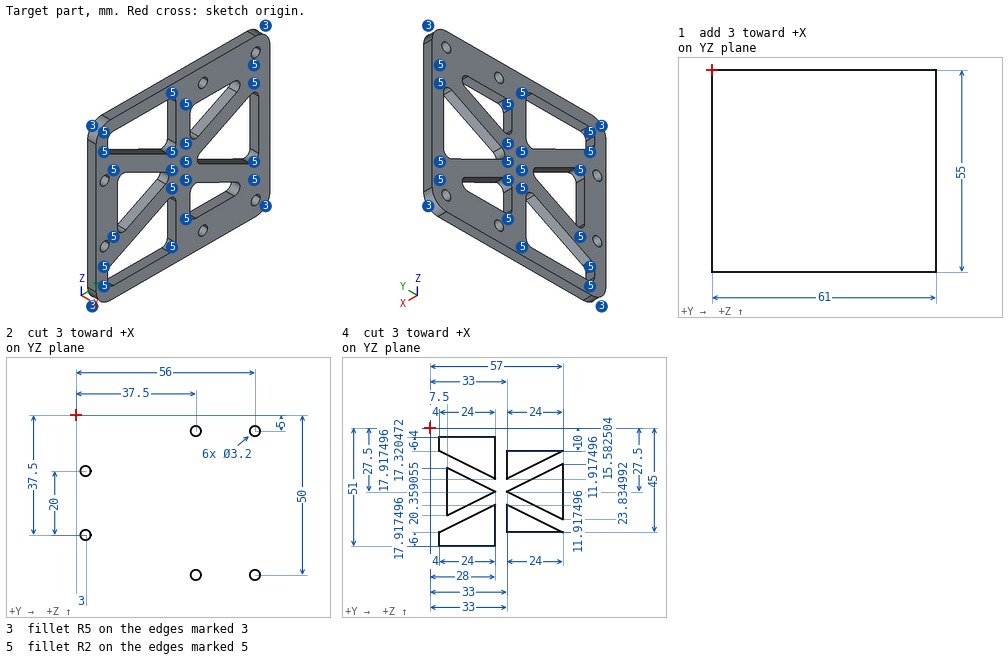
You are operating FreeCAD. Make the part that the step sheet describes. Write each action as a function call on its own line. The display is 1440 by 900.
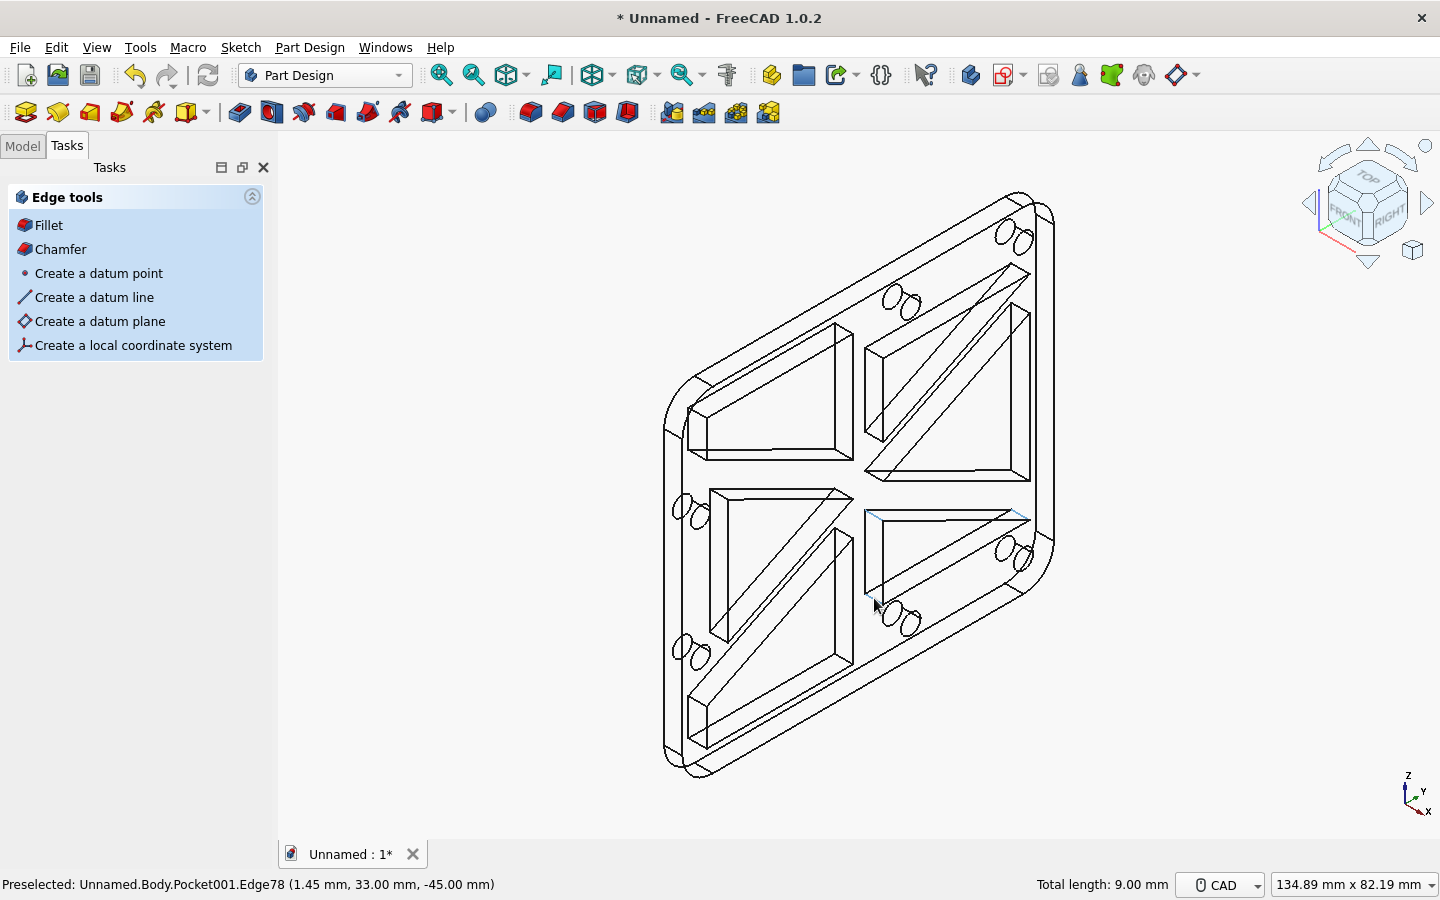
click(1017, 473, ctrl)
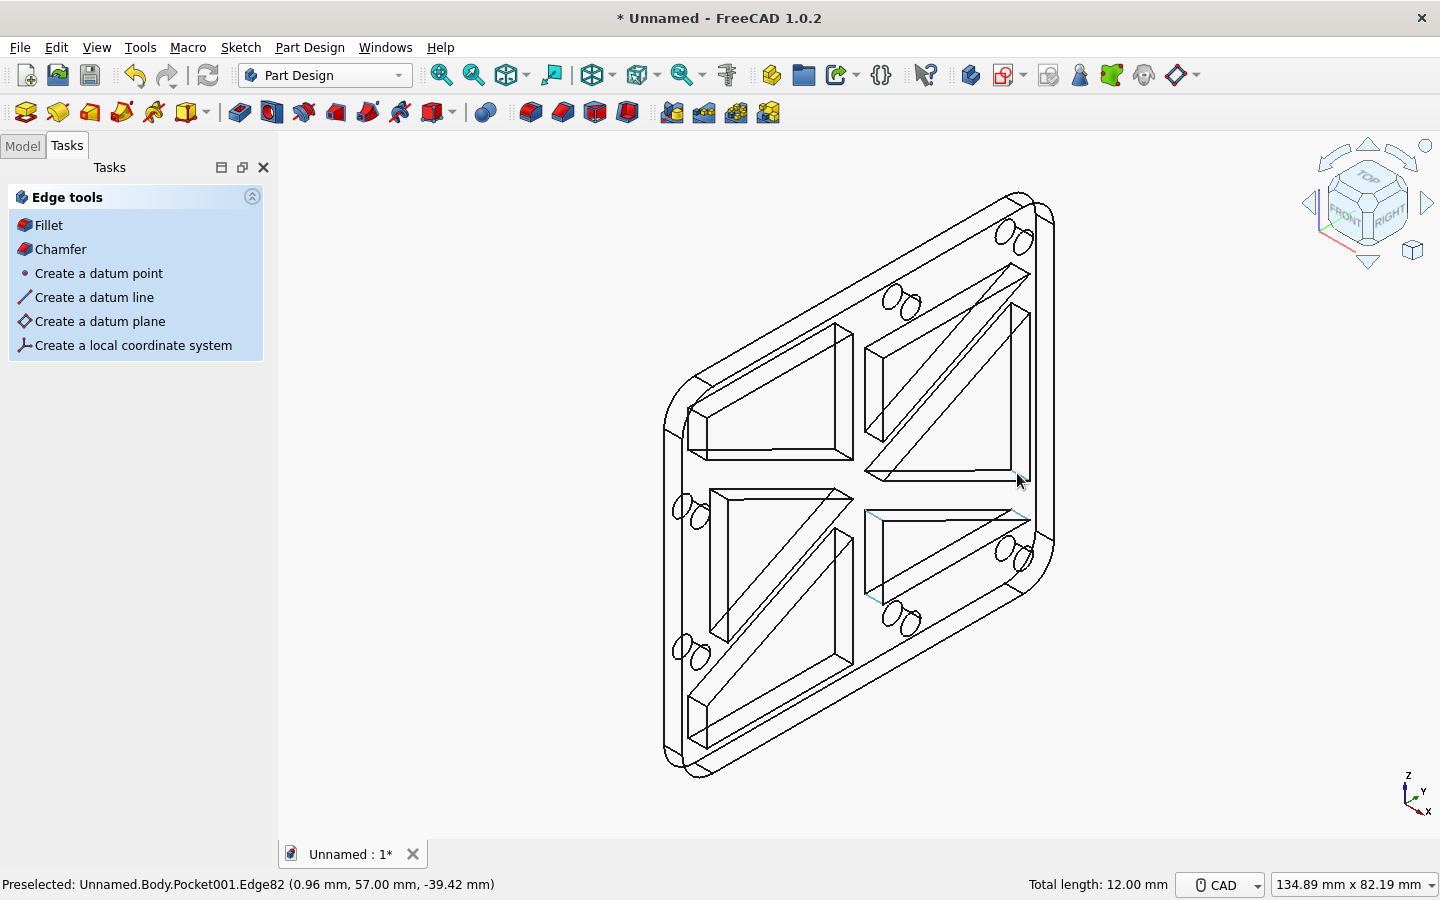
click(1020, 307, ctrl)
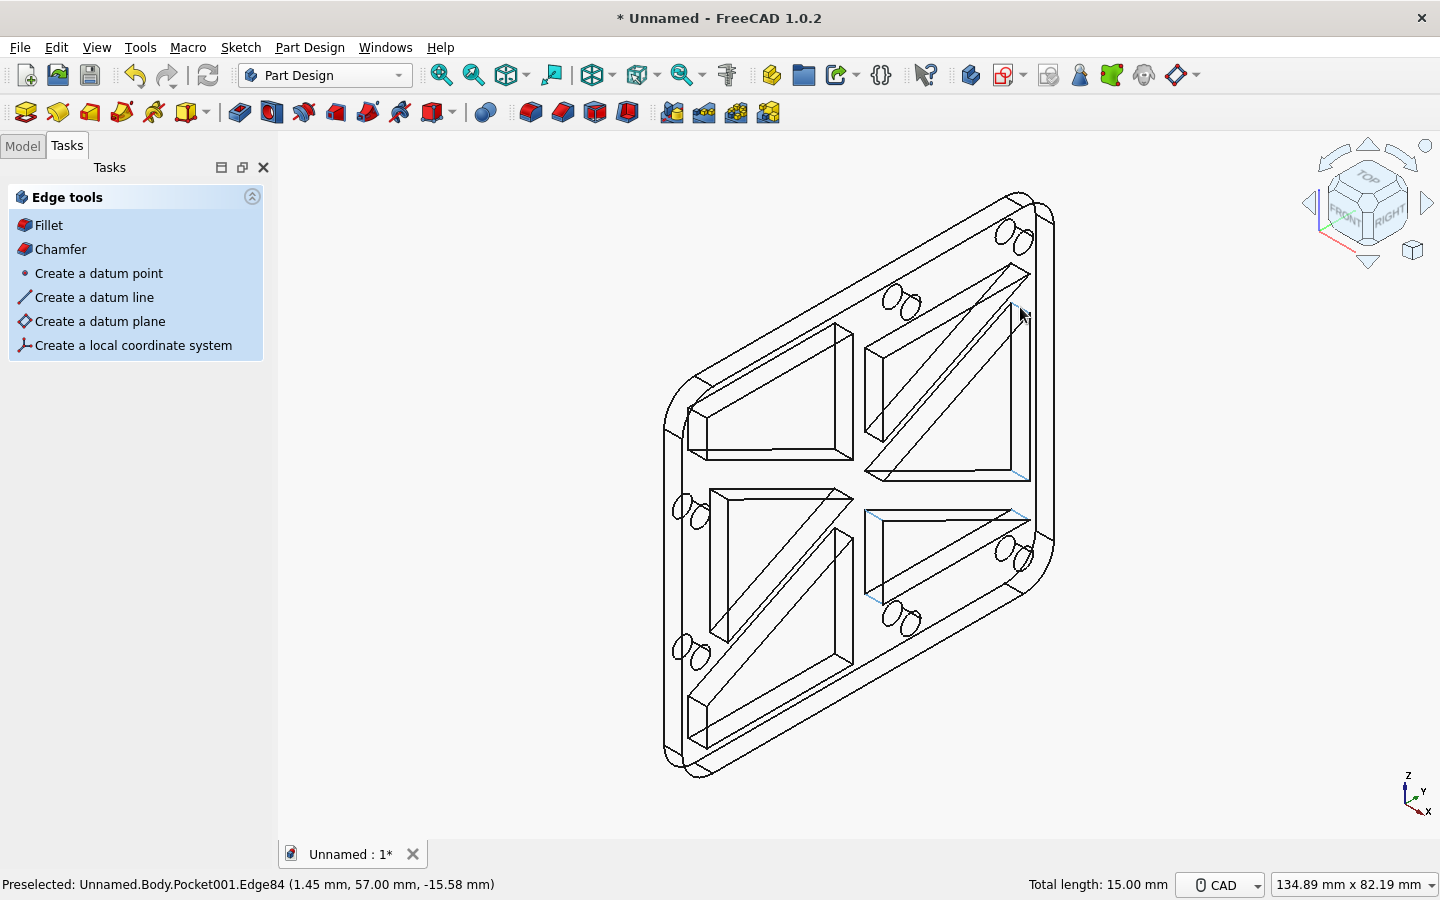
click(874, 475, ctrl)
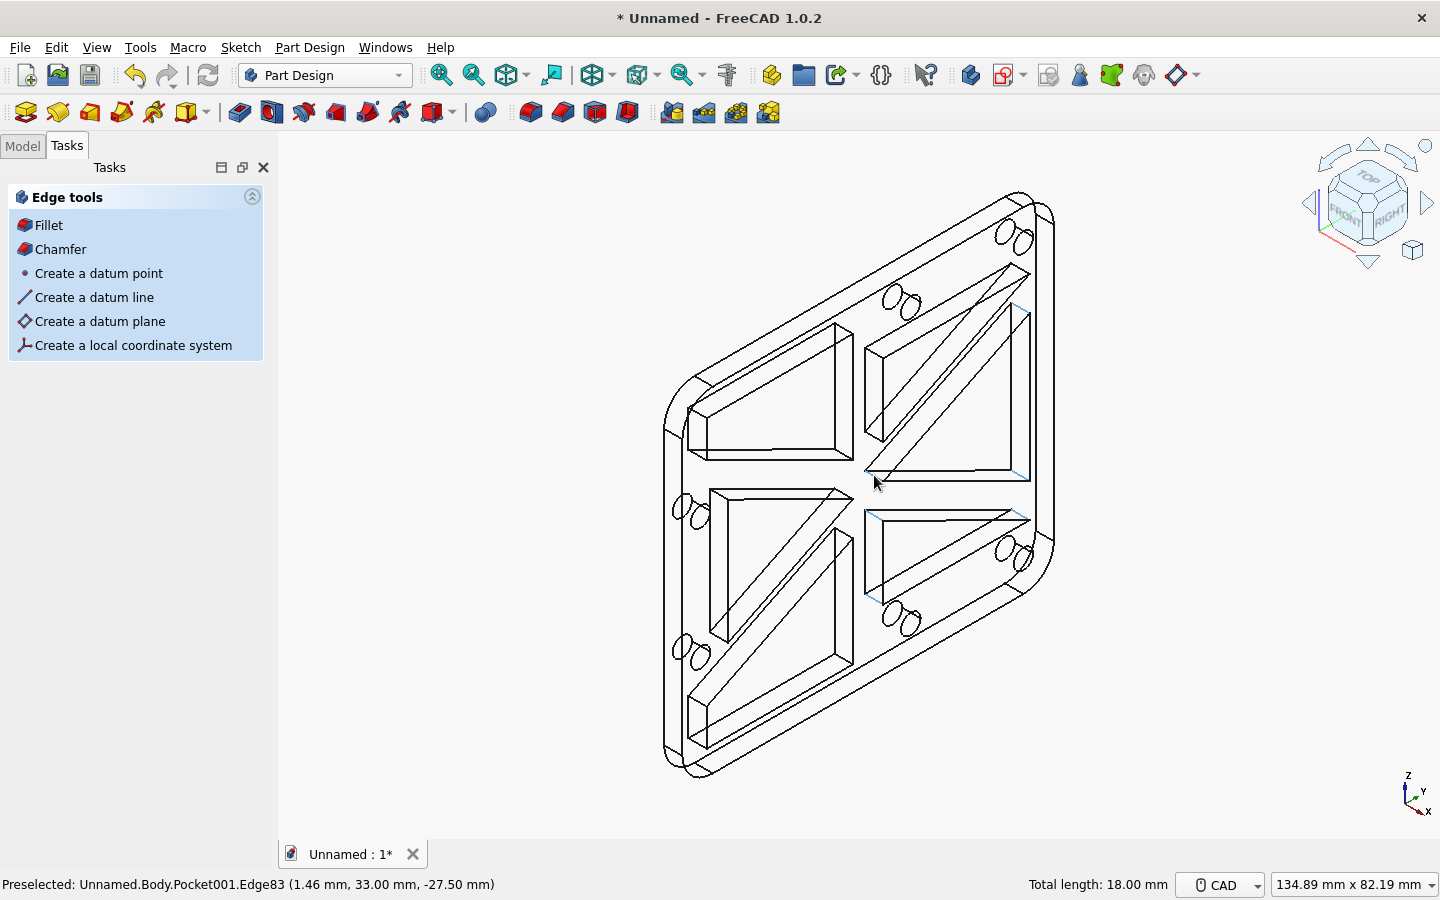
click(842, 492, ctrl)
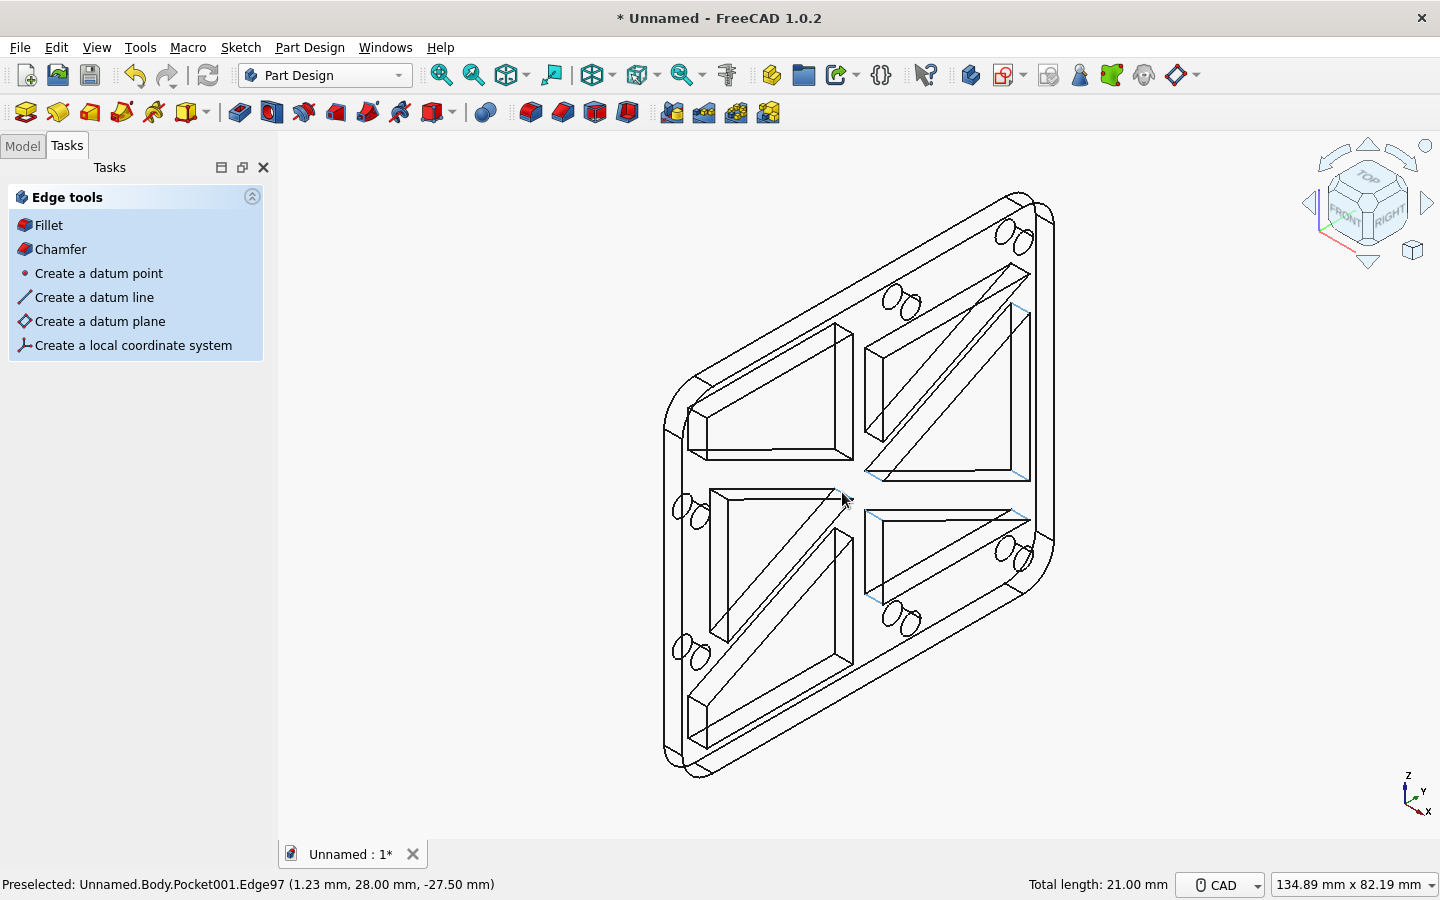
click(719, 493, ctrl)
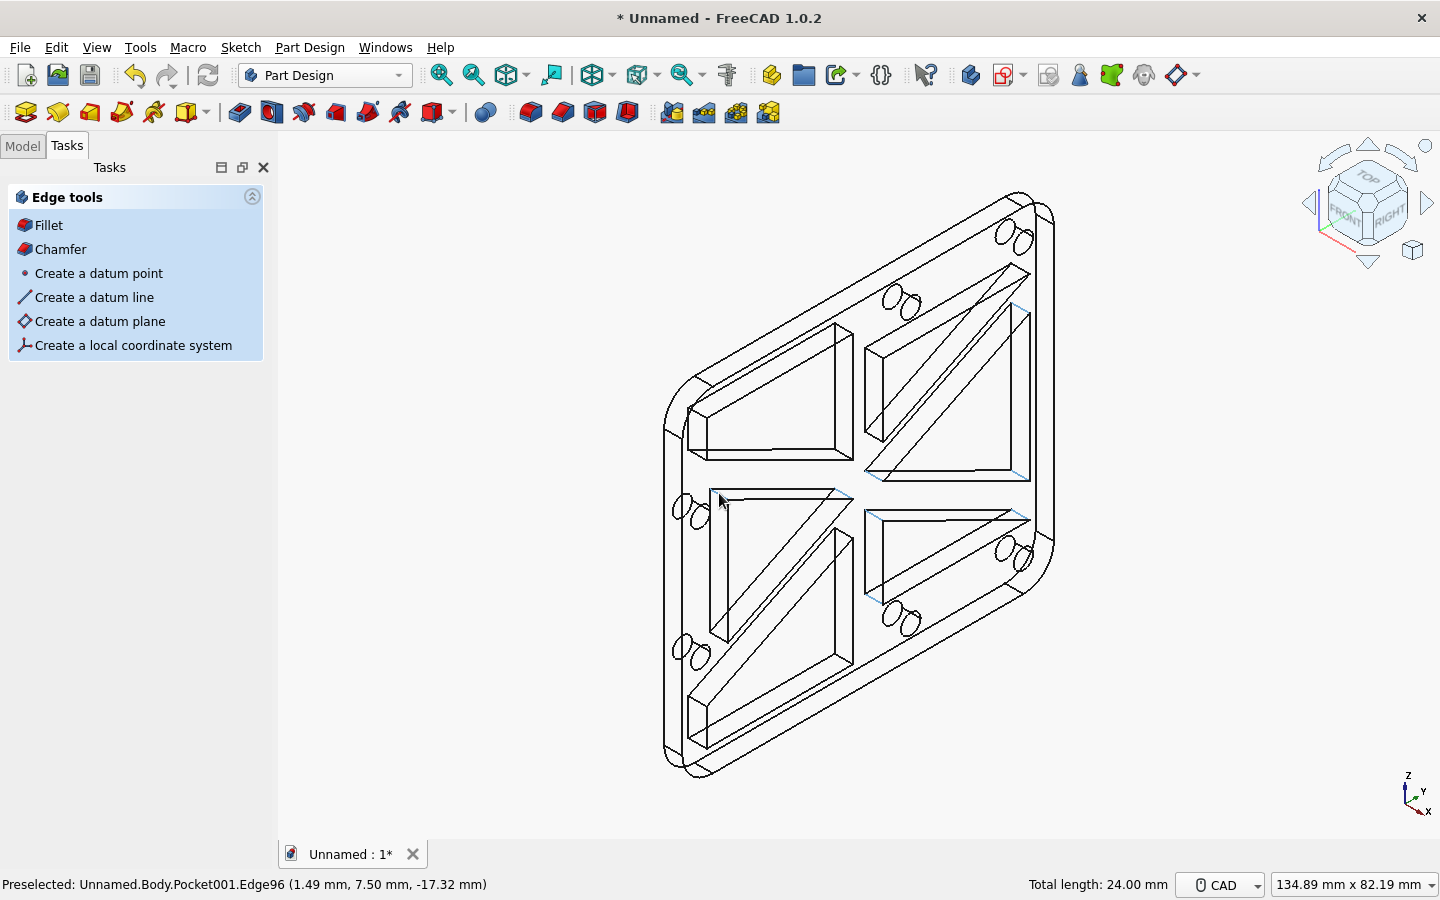
click(719, 636, ctrl)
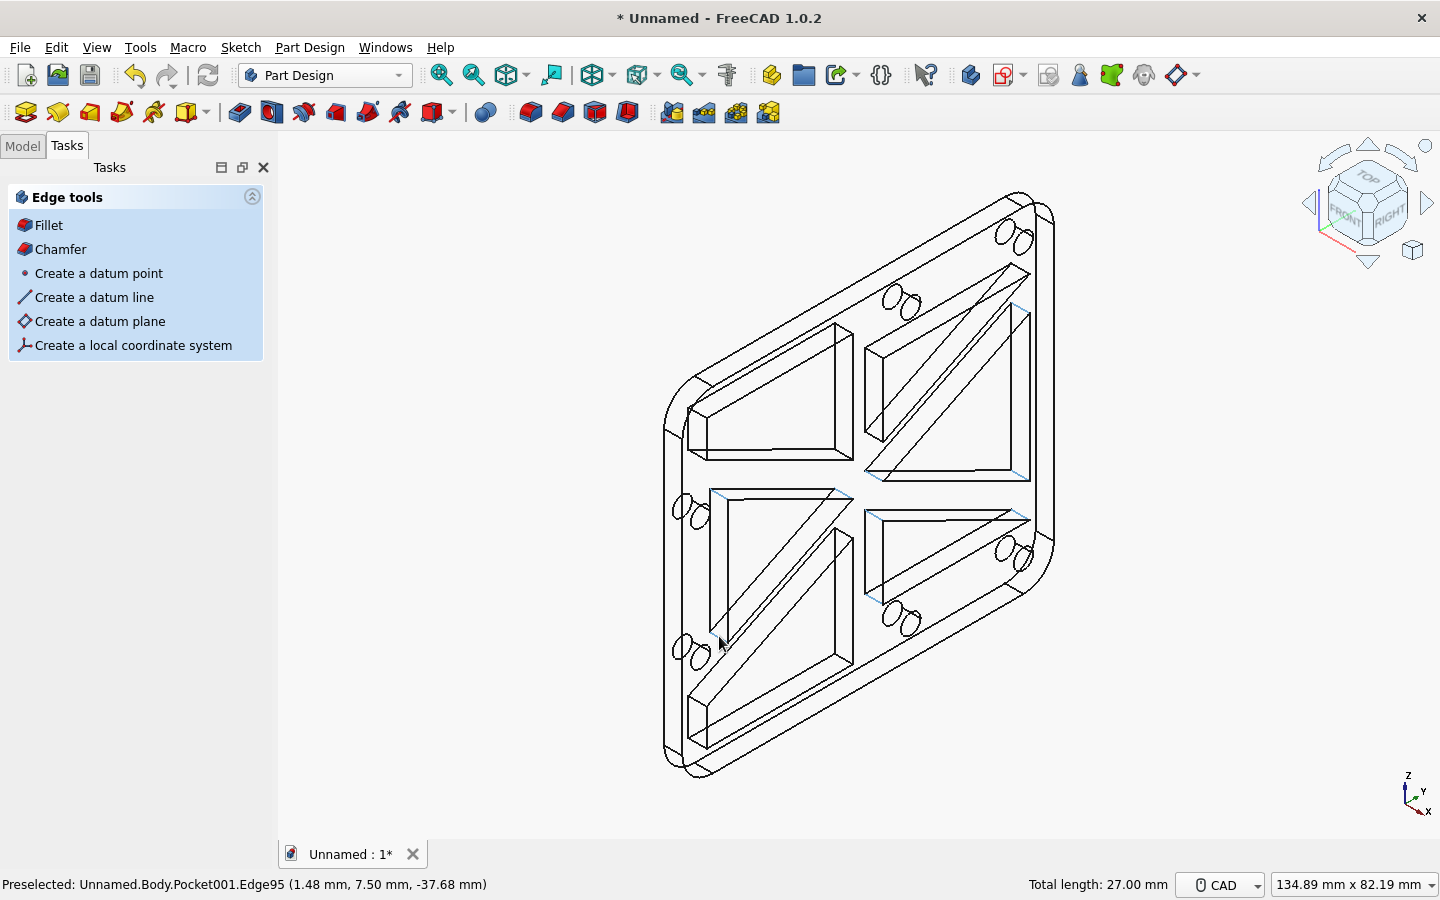
click(844, 328, ctrl)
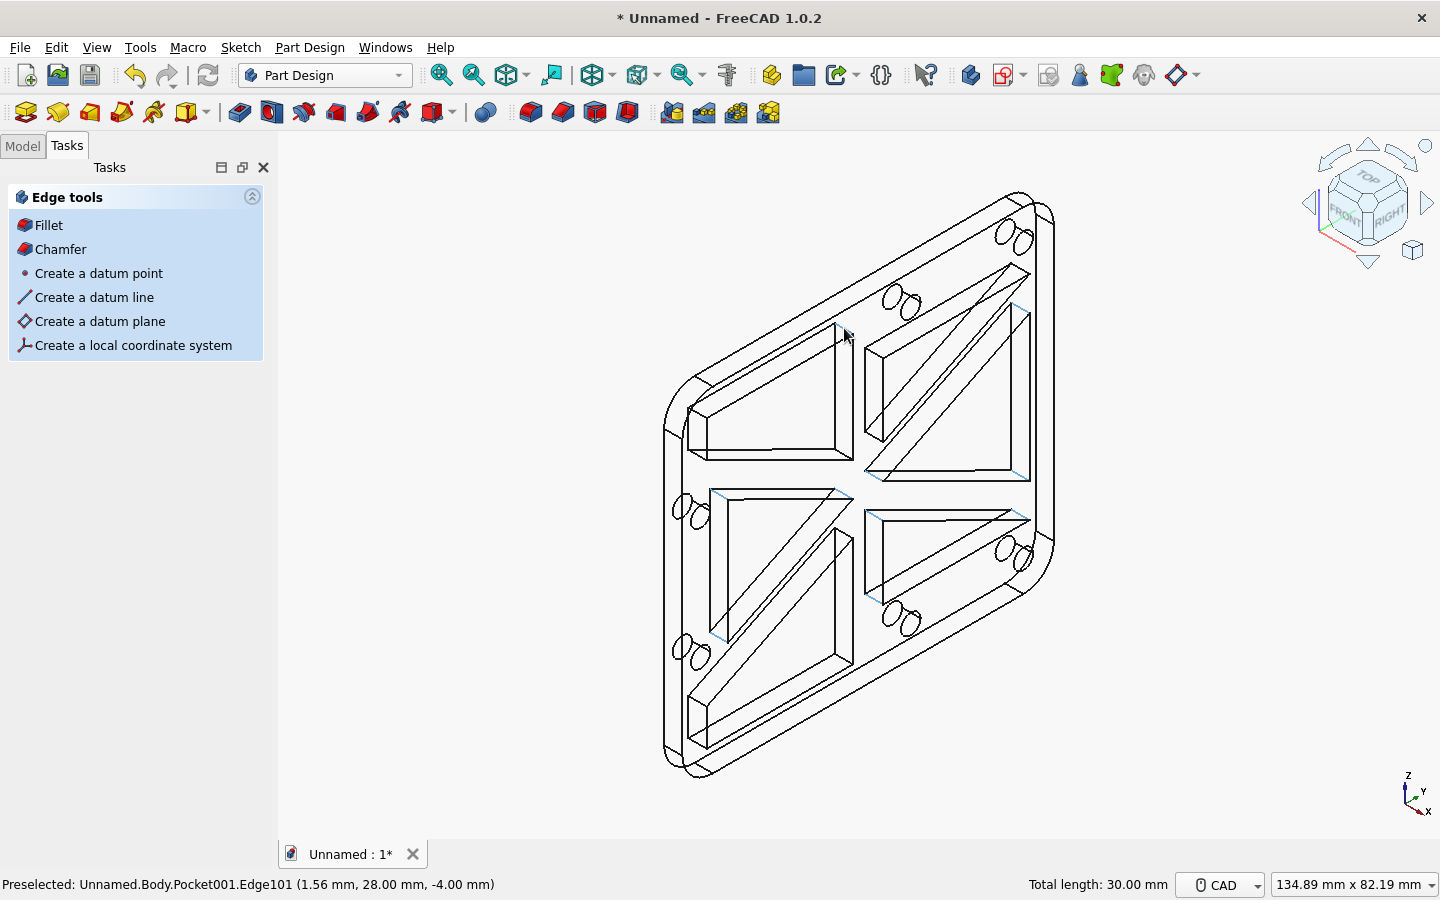
click(698, 412, ctrl)